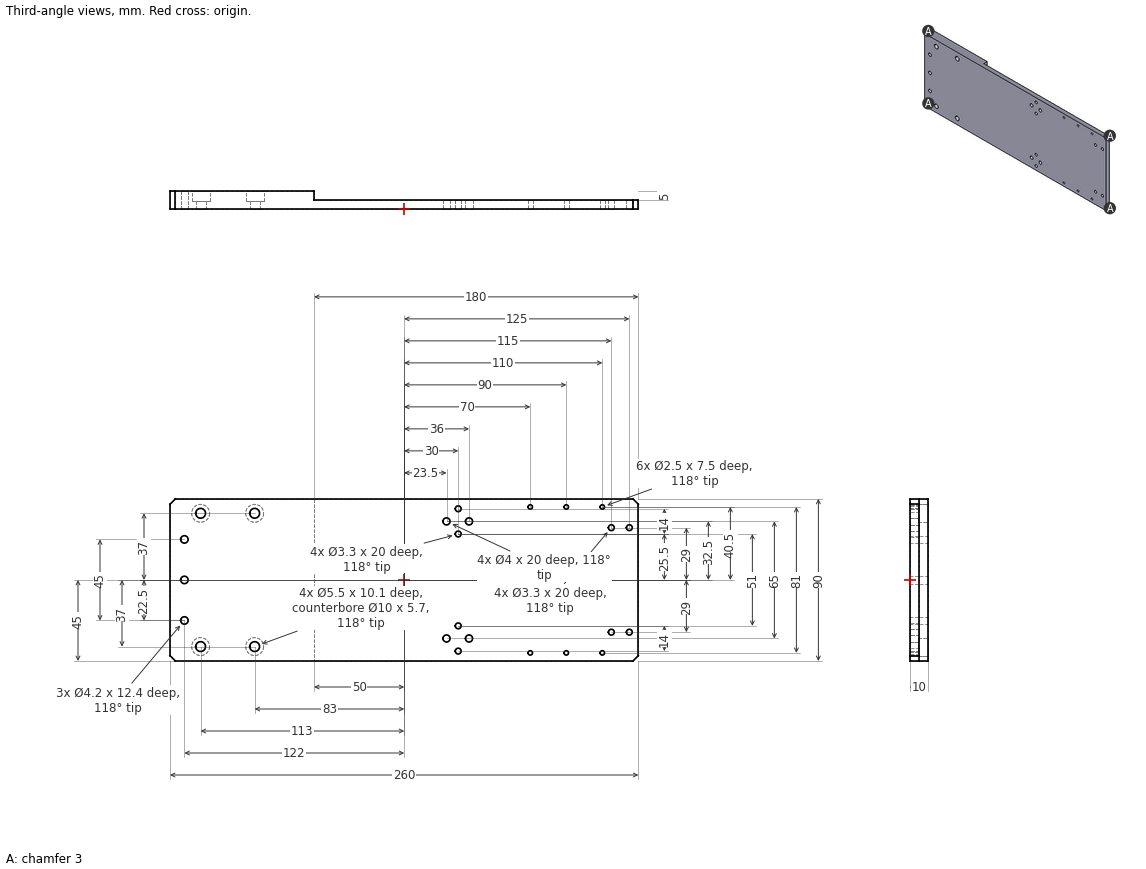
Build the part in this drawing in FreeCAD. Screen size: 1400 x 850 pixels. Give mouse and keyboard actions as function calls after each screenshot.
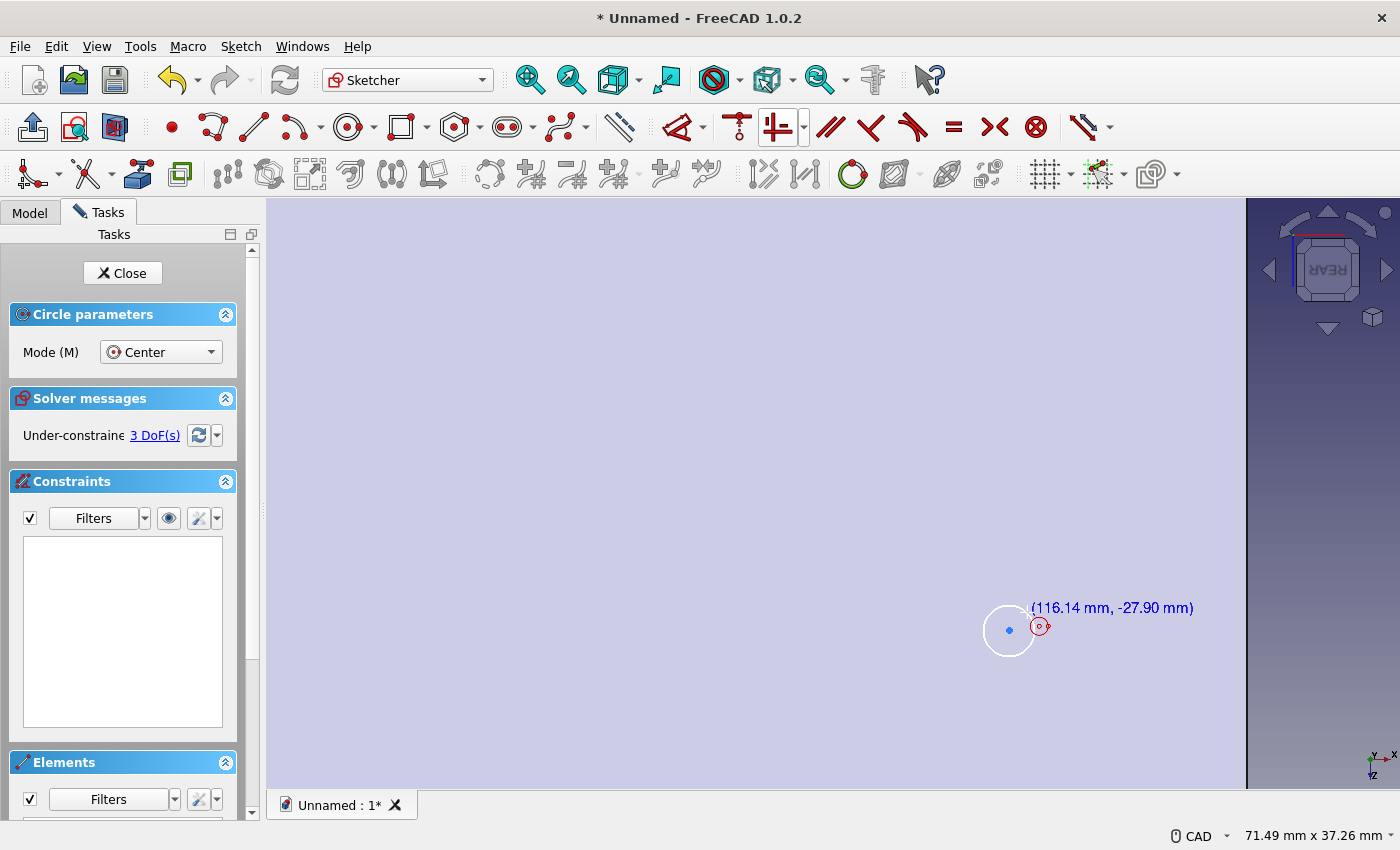
click(1167, 630)
click(1186, 612)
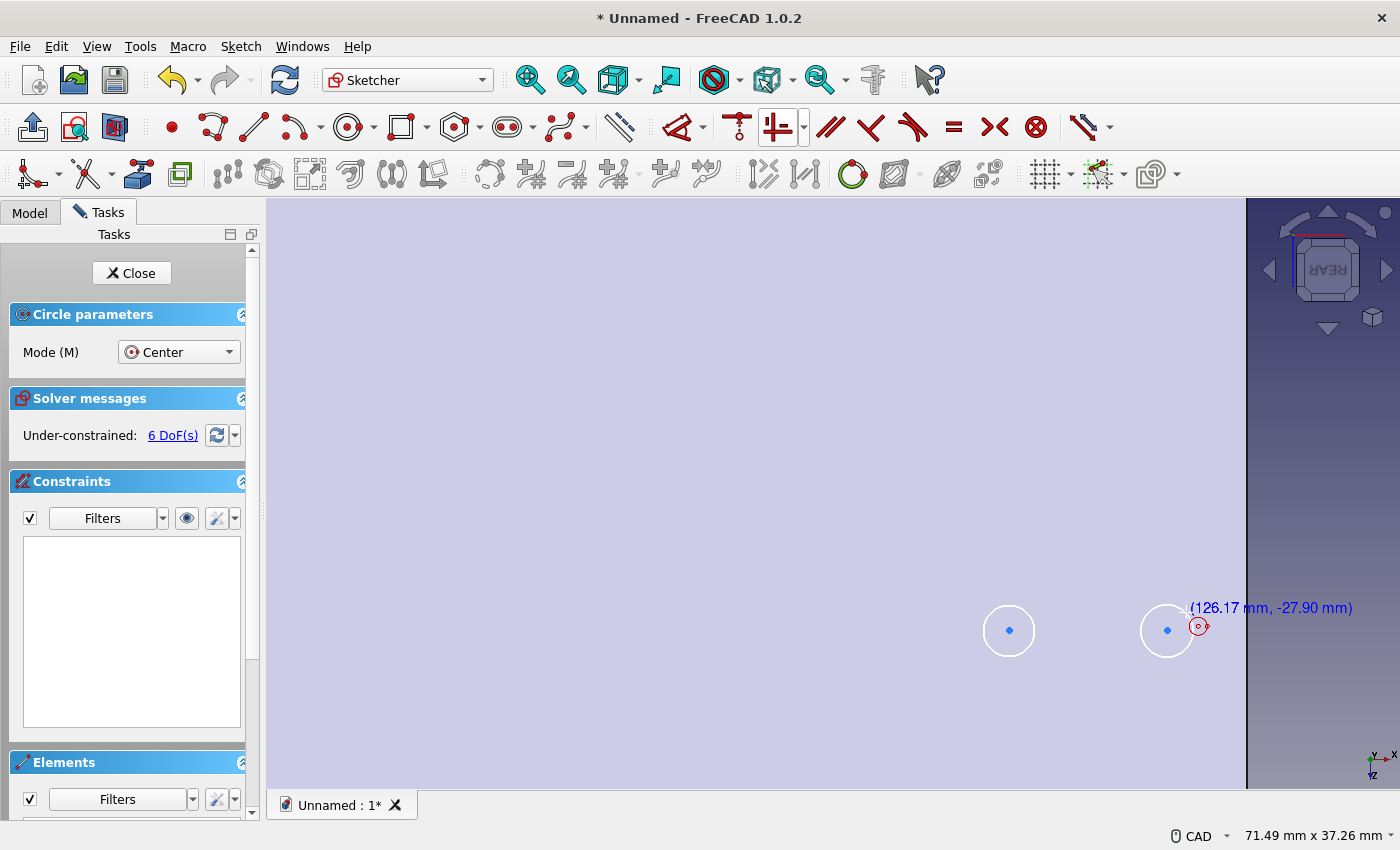
scroll(1012, 633, down, 6)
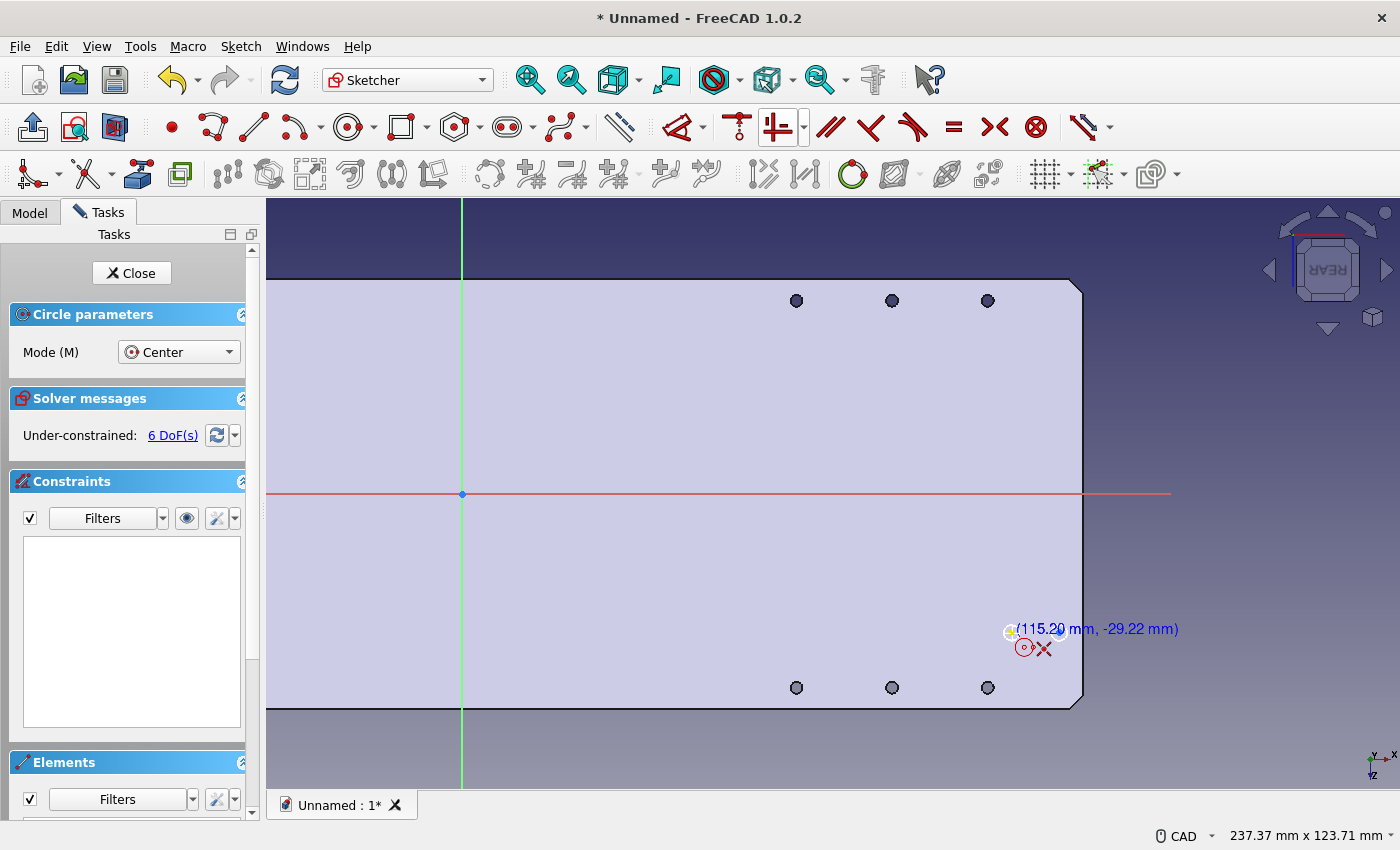
scroll(1012, 356, up, 6)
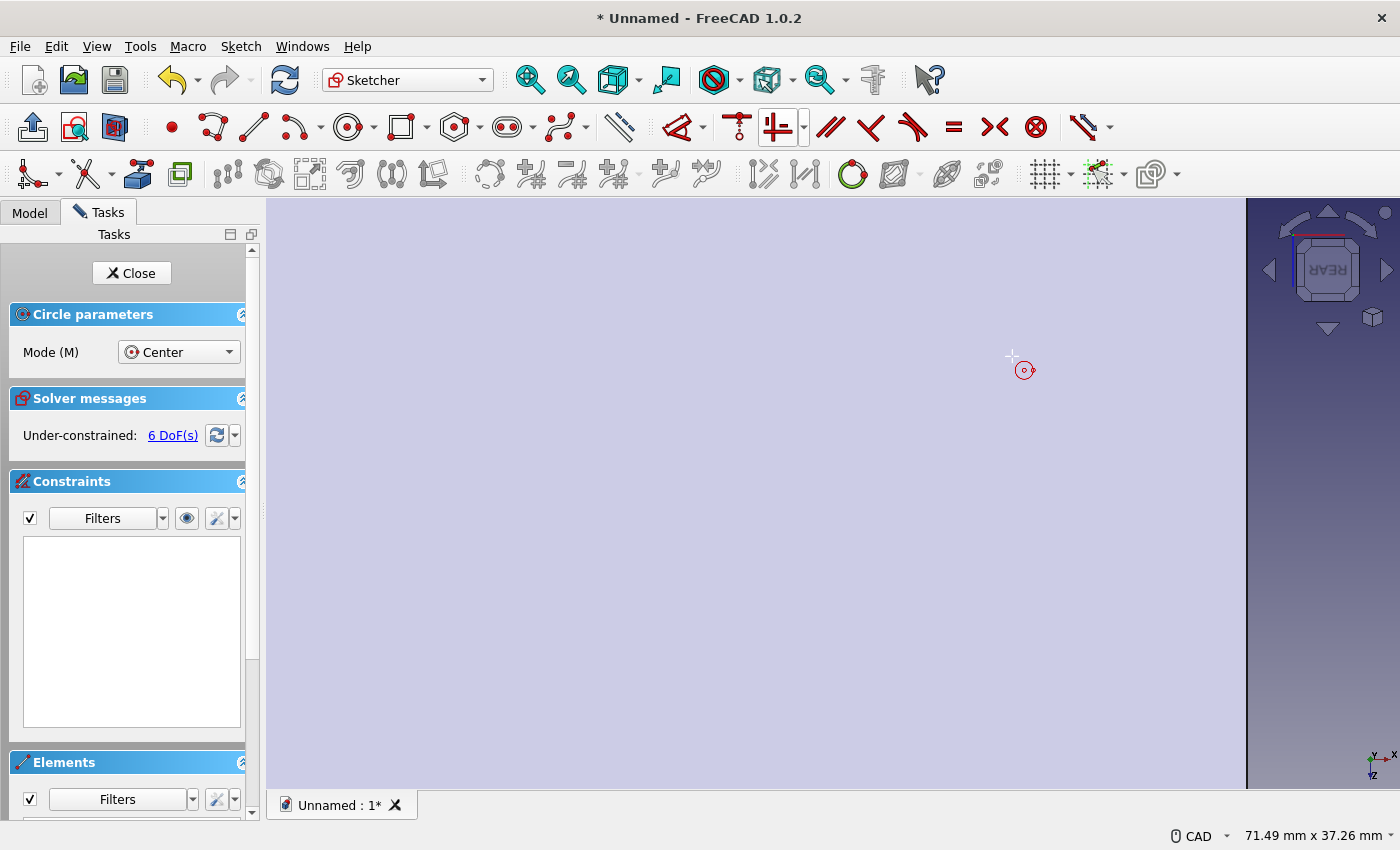
click(1009, 354)
click(1027, 336)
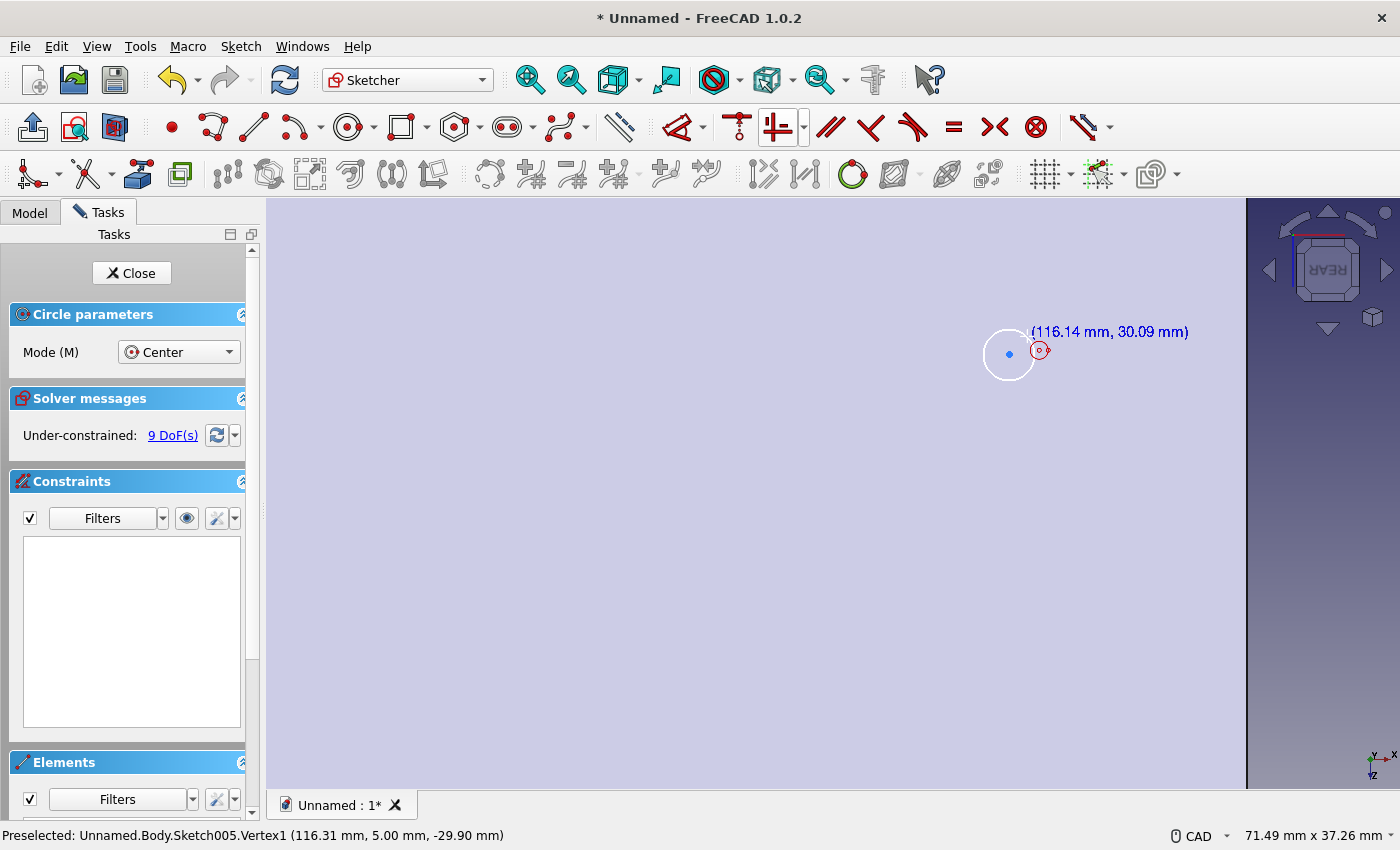
click(1167, 354)
click(1186, 336)
key(Escape)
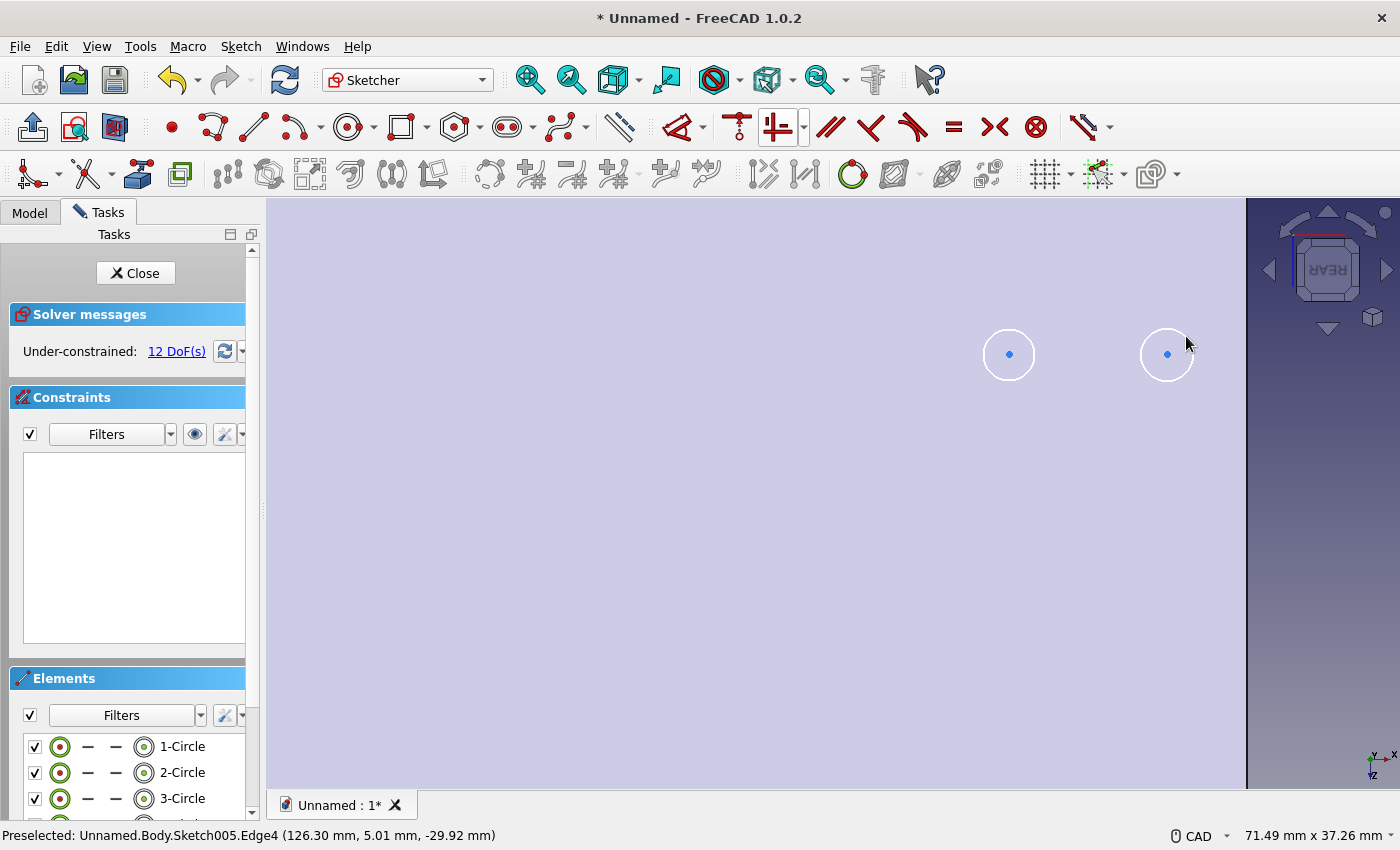
scroll(1012, 355, down, 6)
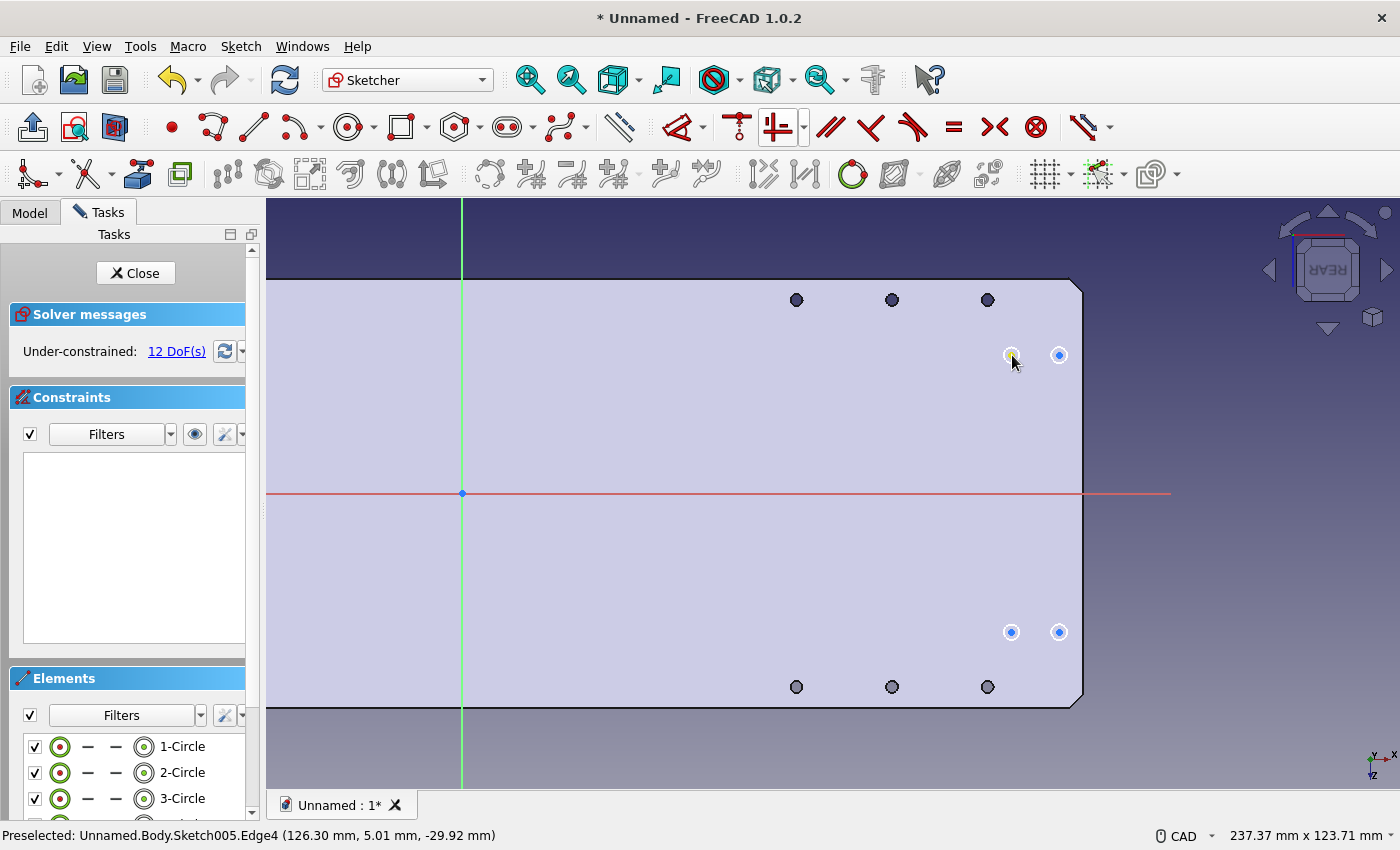
scroll(1017, 627, up, 3)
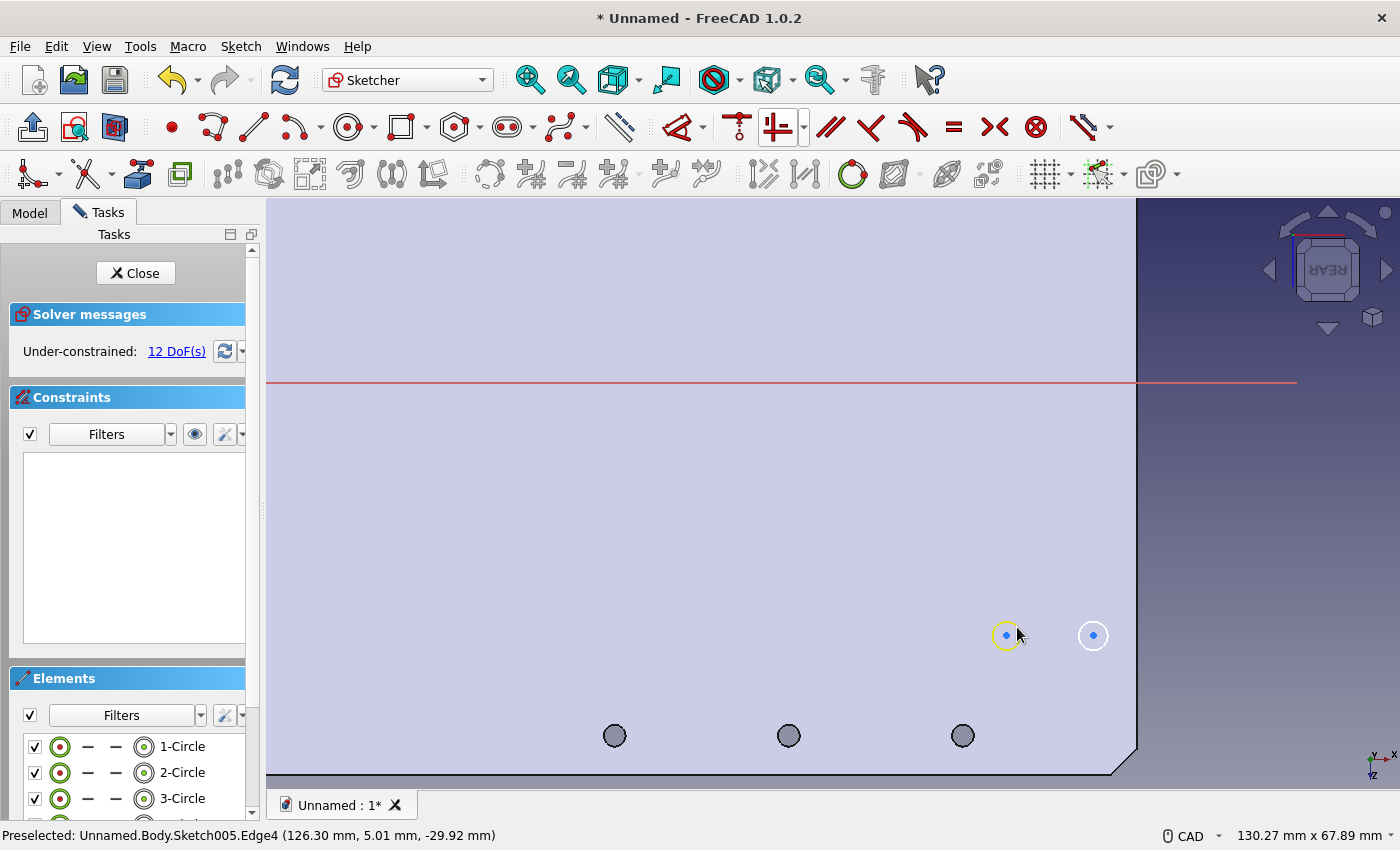
click(1016, 626)